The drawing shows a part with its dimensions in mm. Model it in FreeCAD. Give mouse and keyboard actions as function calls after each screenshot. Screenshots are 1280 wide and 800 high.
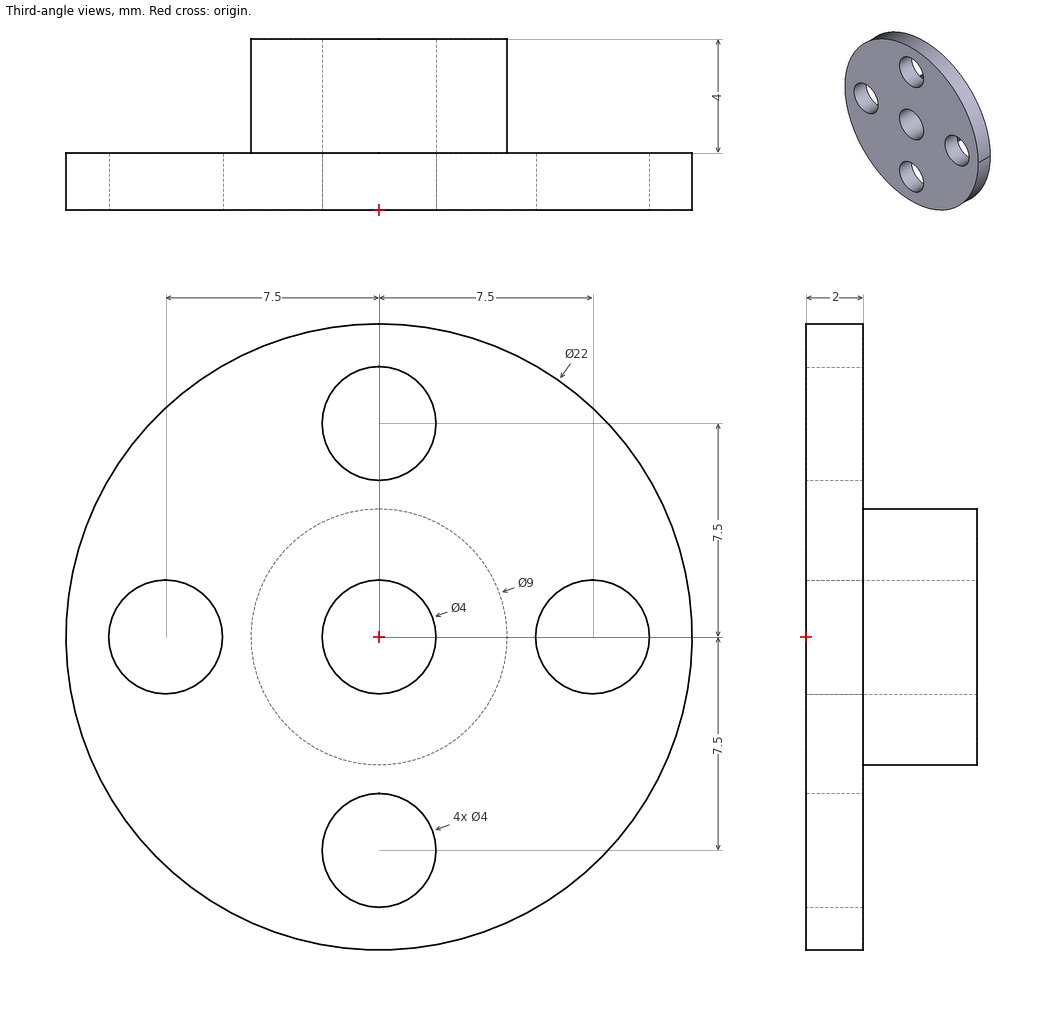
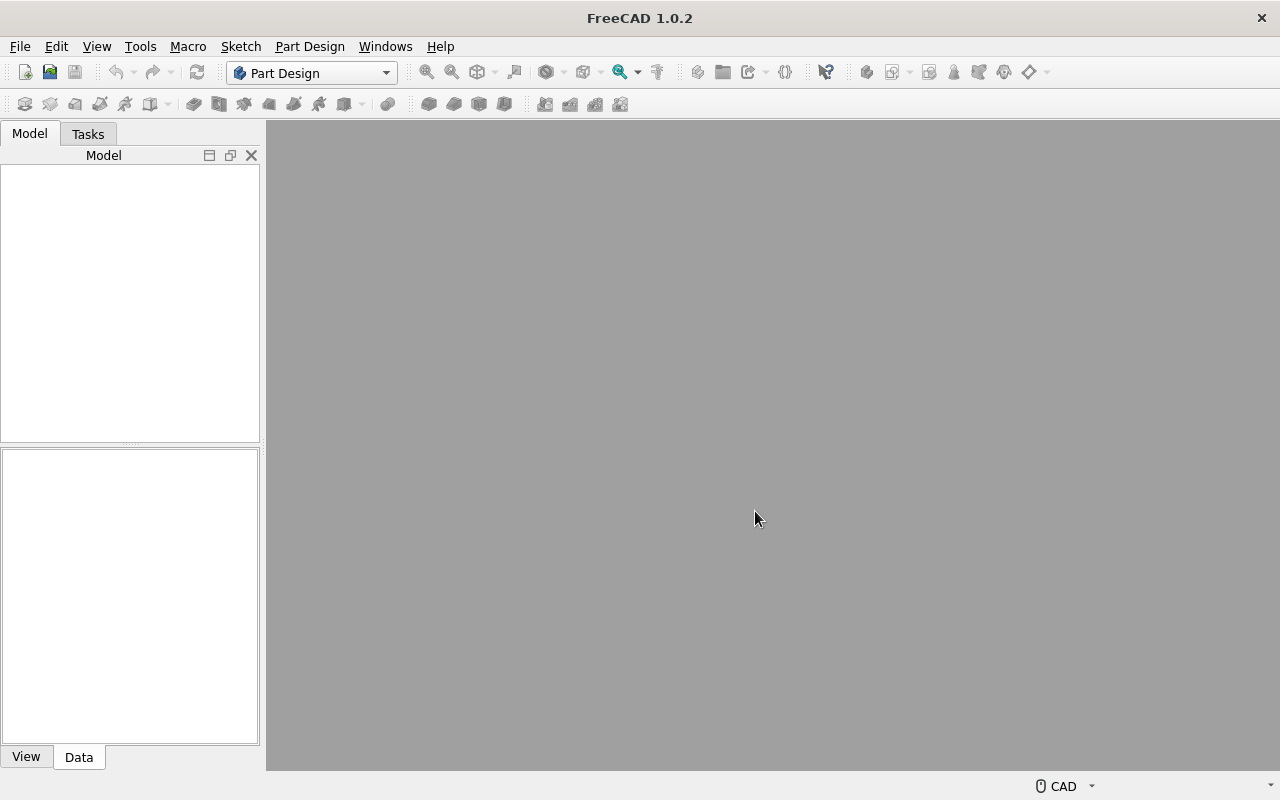
click(25, 72)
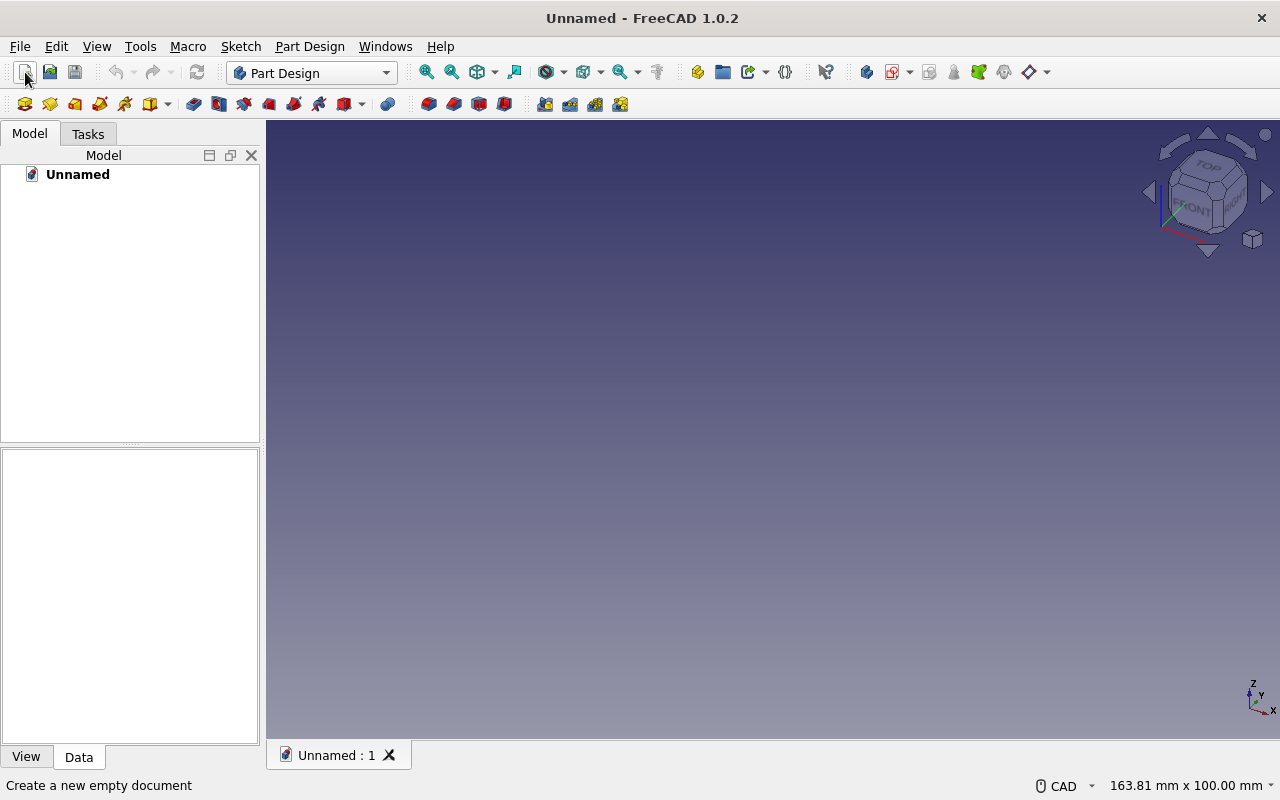
click(892, 72)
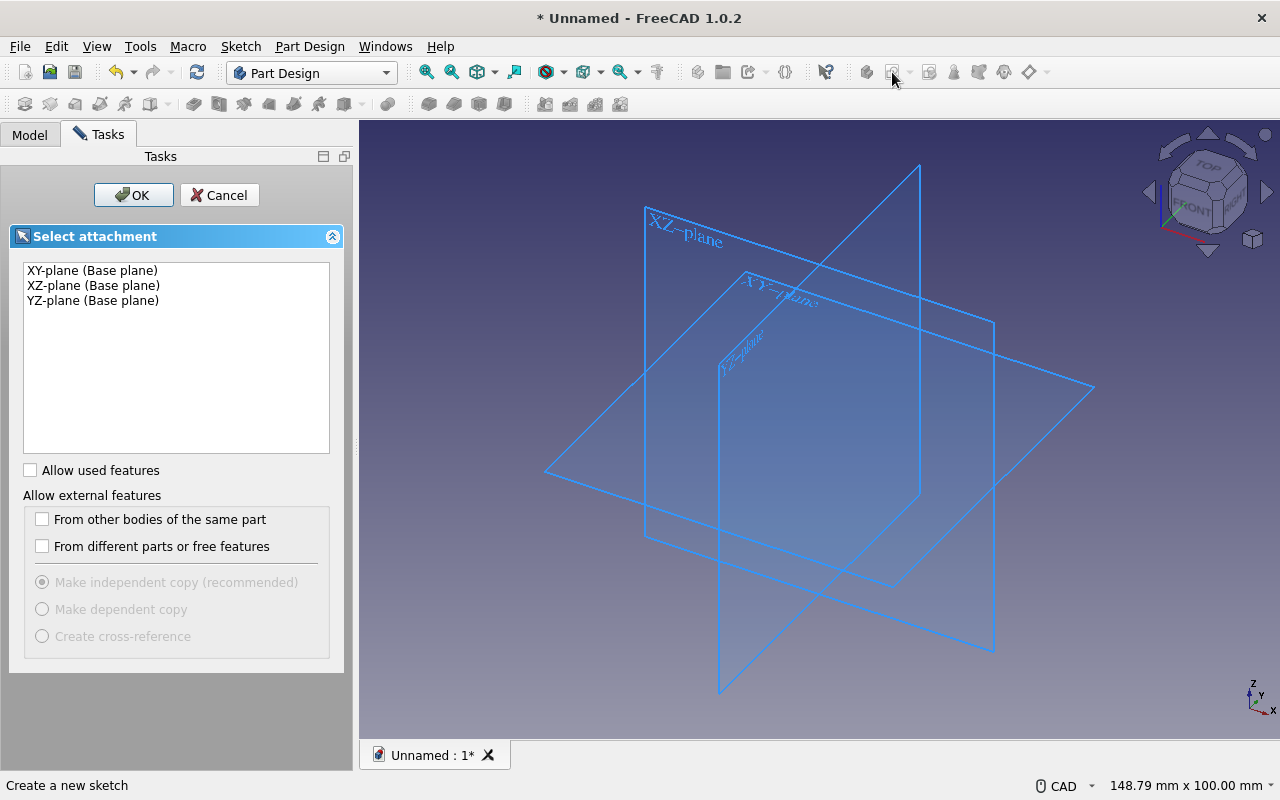
click(84, 286)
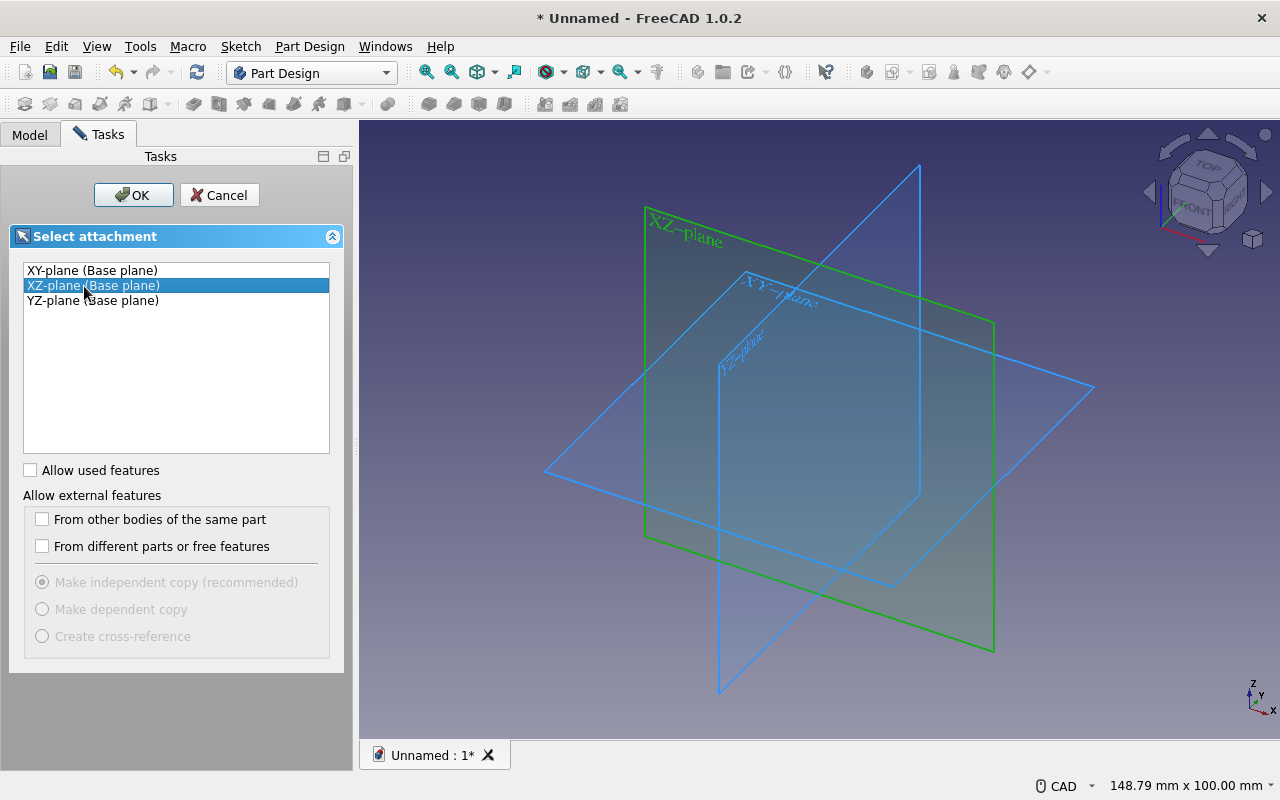
click(134, 195)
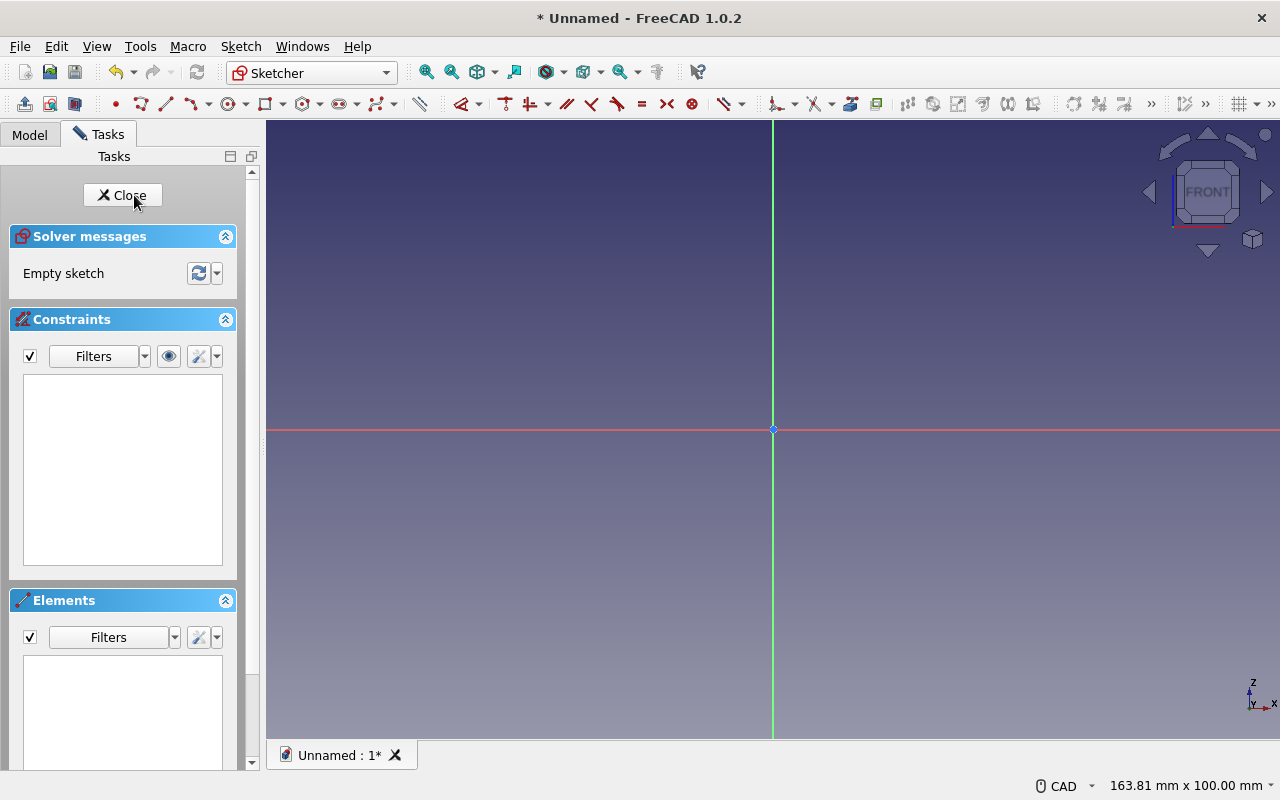
scroll(813, 429, up, 5)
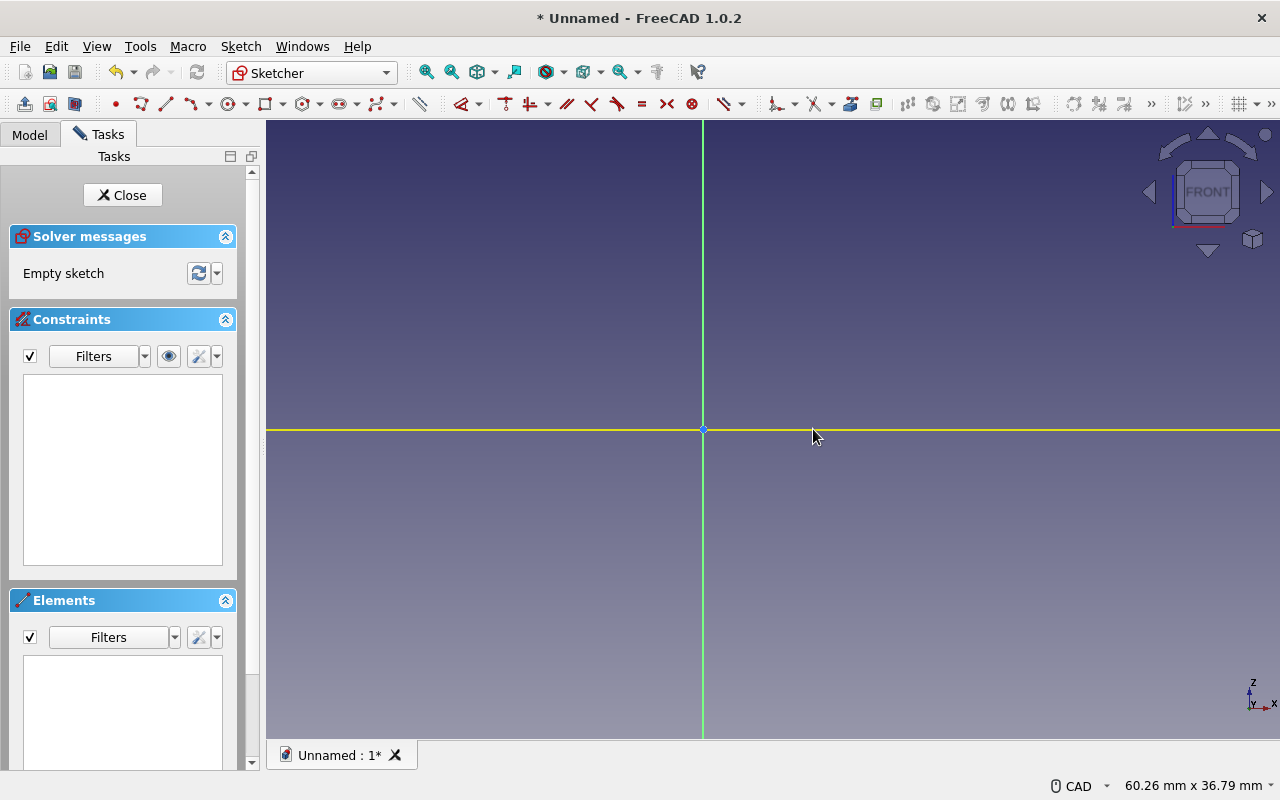
click(228, 104)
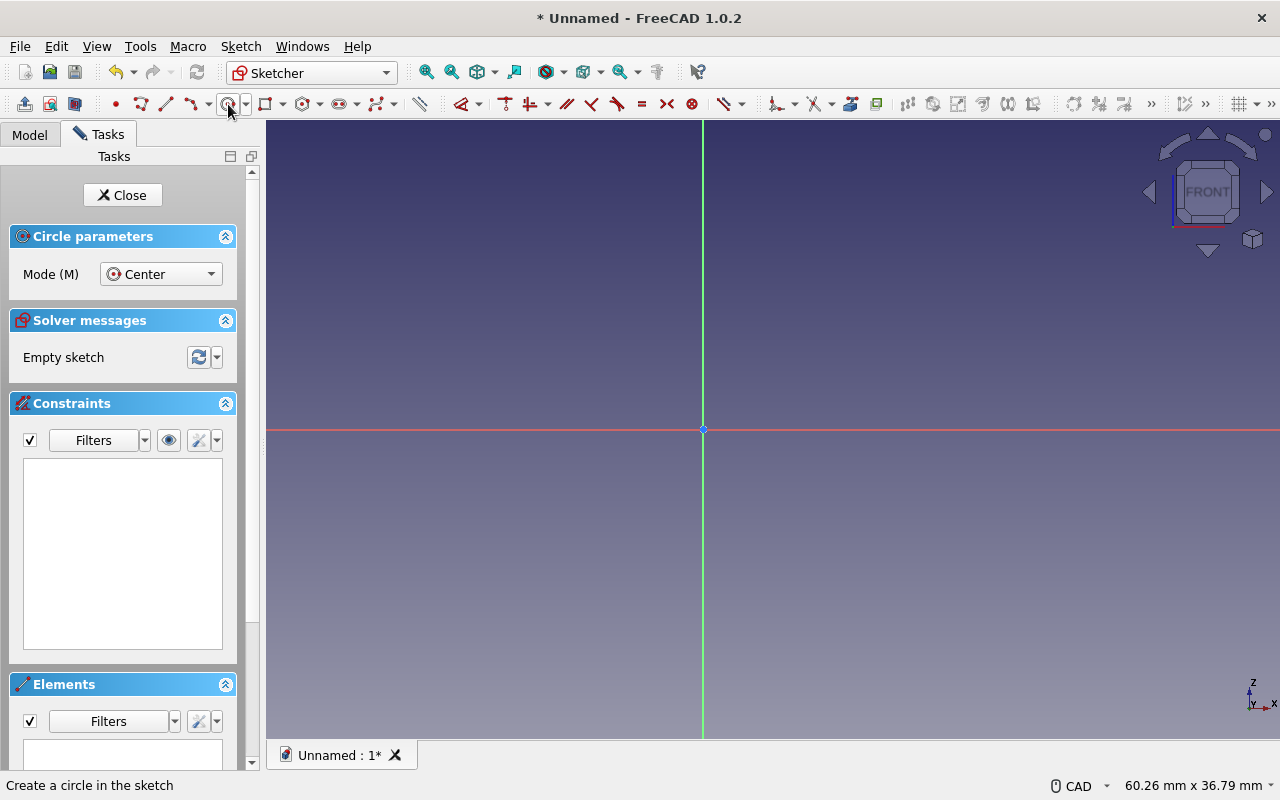
click(703, 430)
click(834, 299)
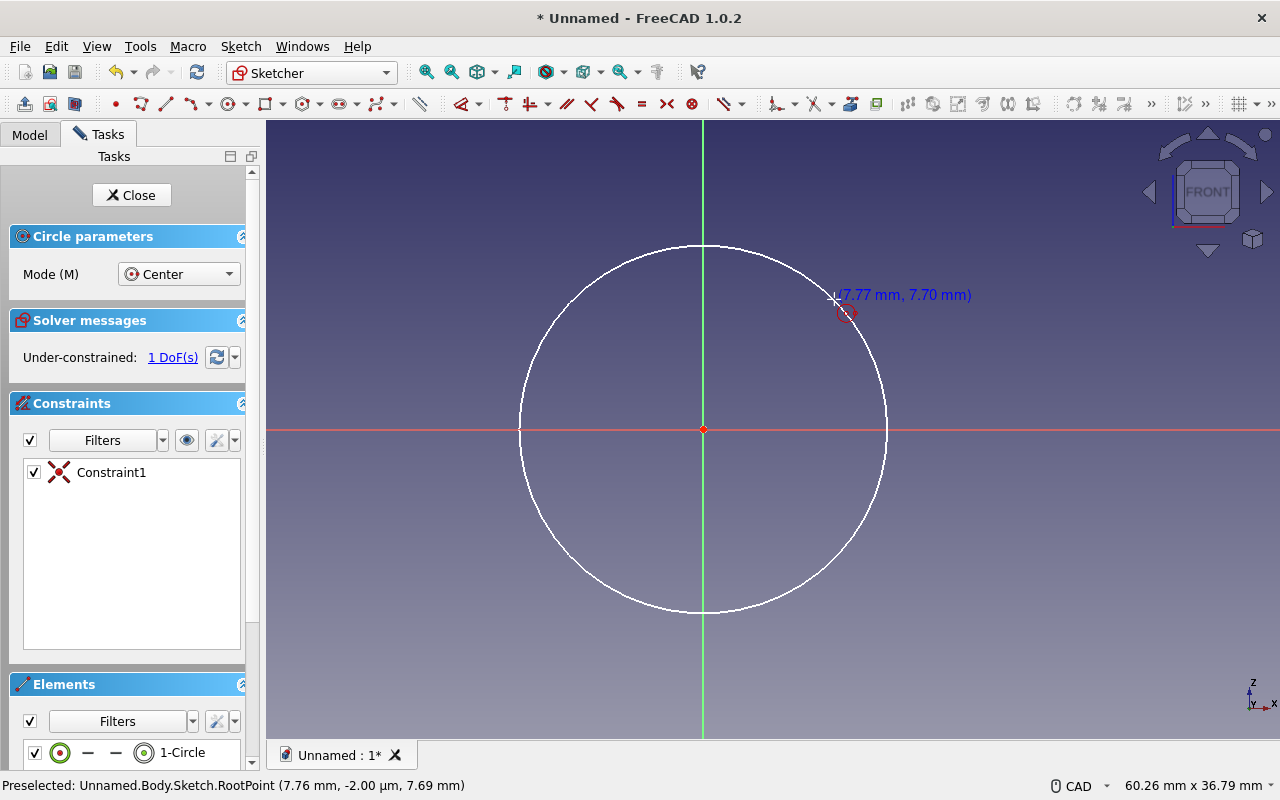
click(703, 556)
click(727, 532)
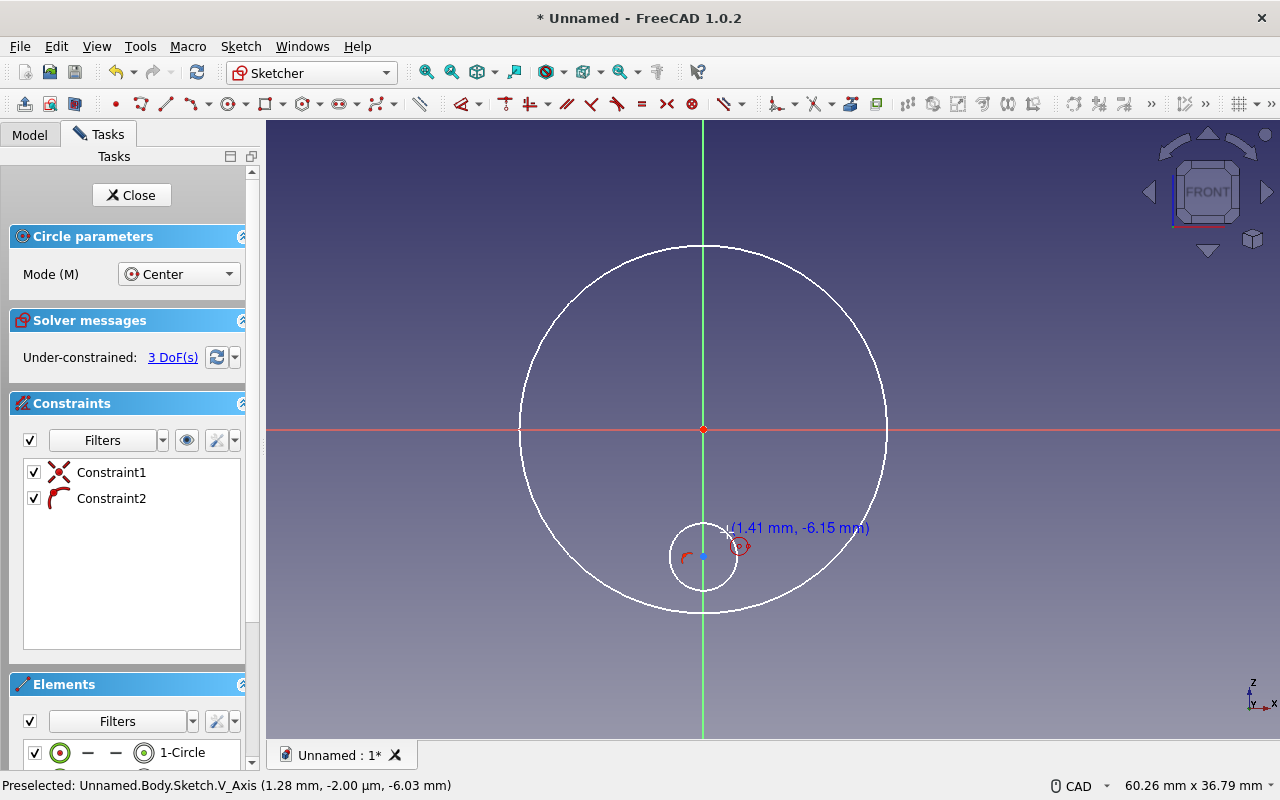
click(577, 430)
click(601, 406)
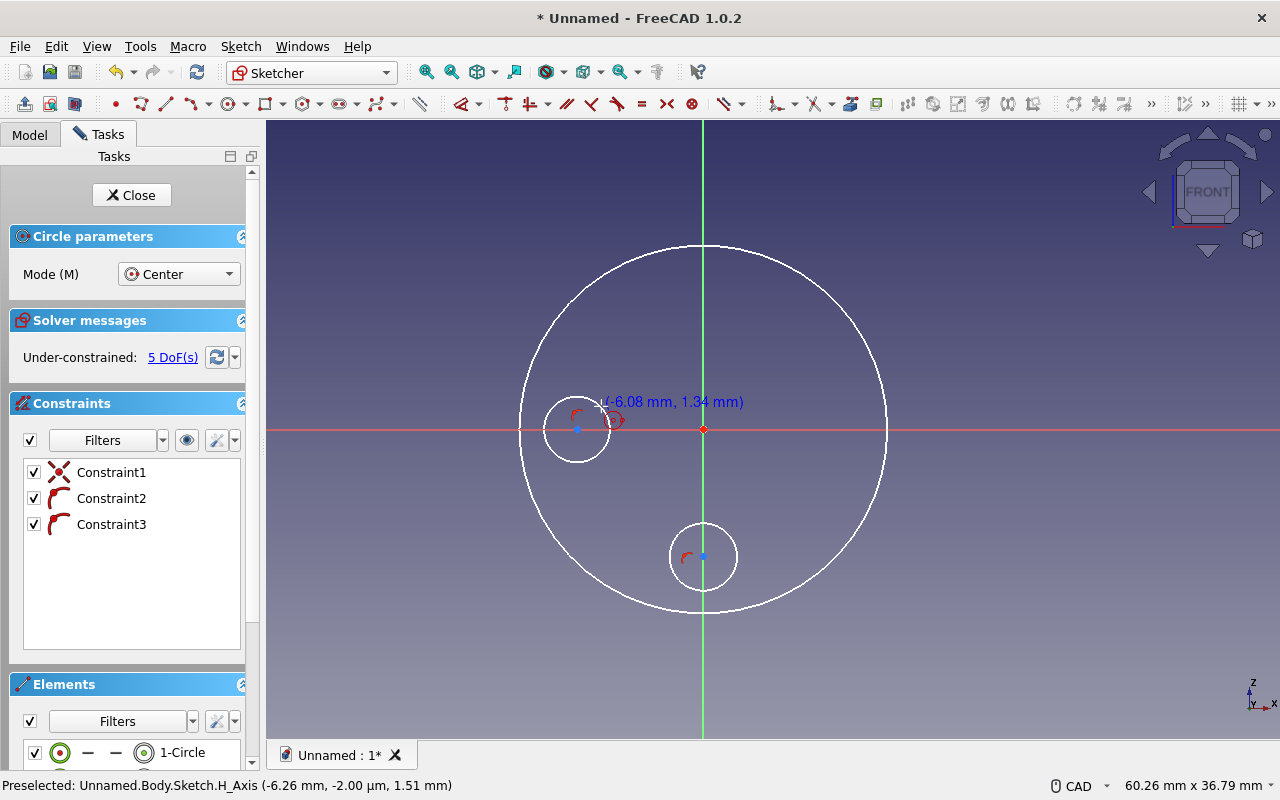
click(703, 303)
click(727, 280)